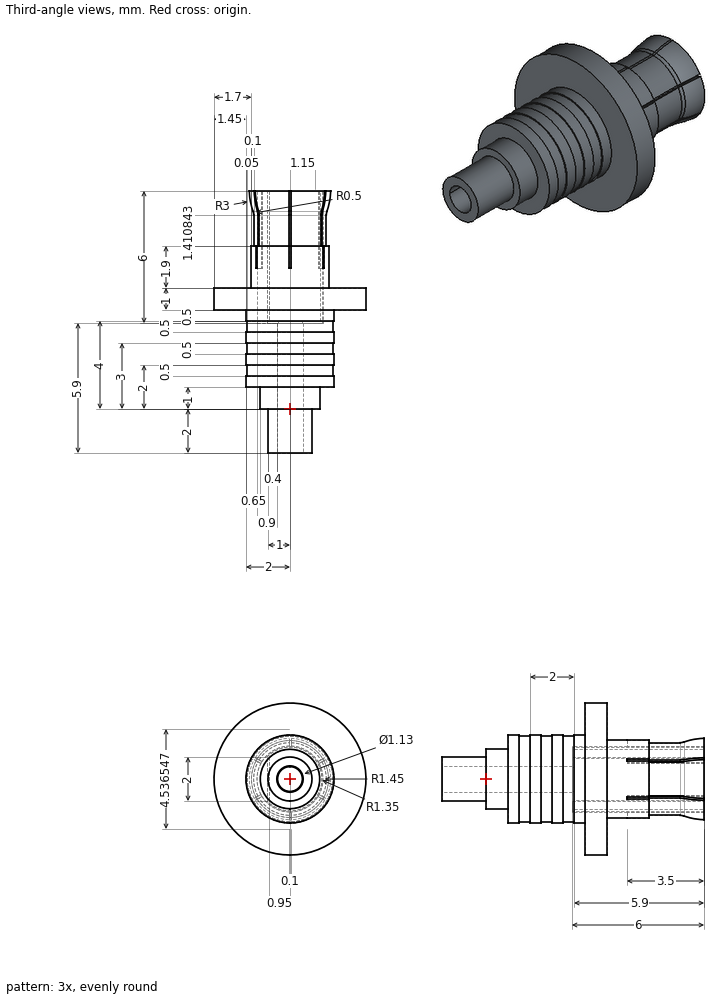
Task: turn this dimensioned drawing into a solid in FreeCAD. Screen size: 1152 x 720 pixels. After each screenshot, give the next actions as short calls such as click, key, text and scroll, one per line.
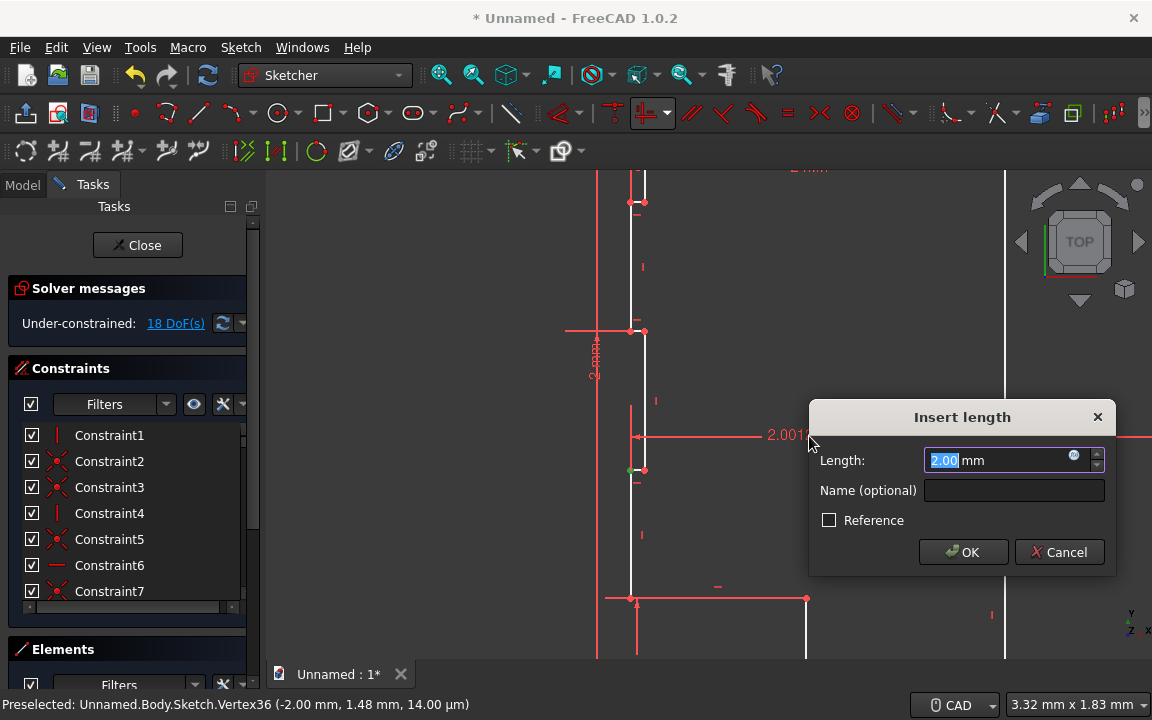
text(2)
key(Return)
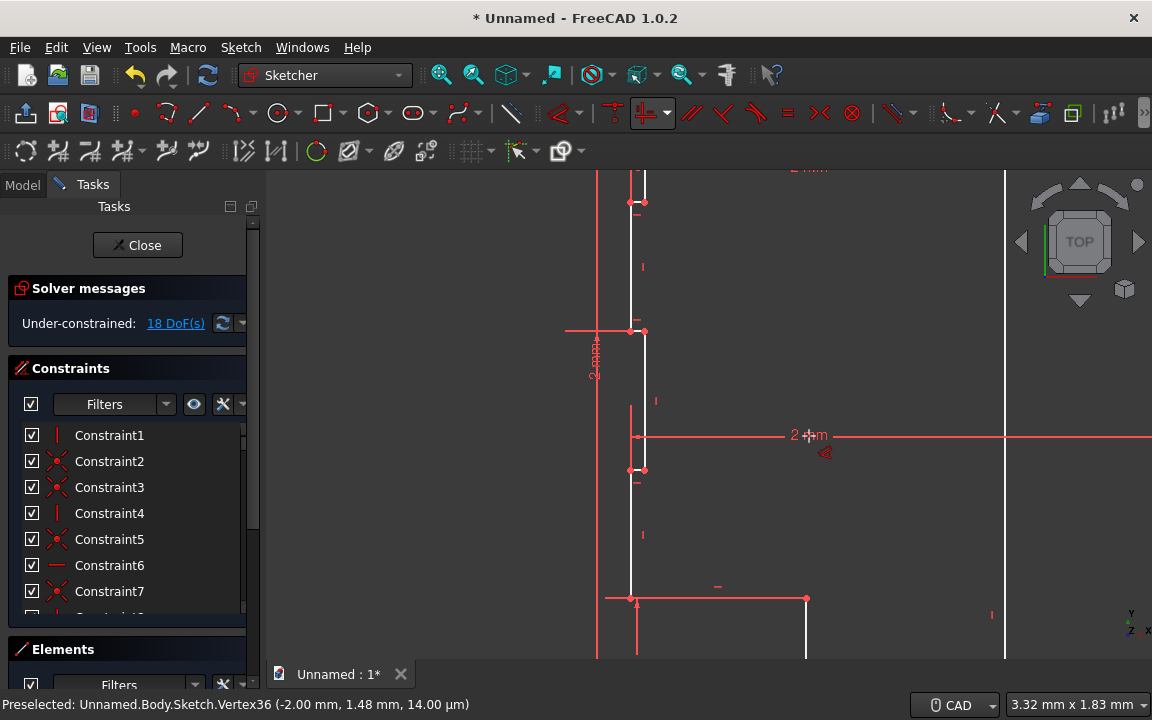
scroll(634, 475, down, 12)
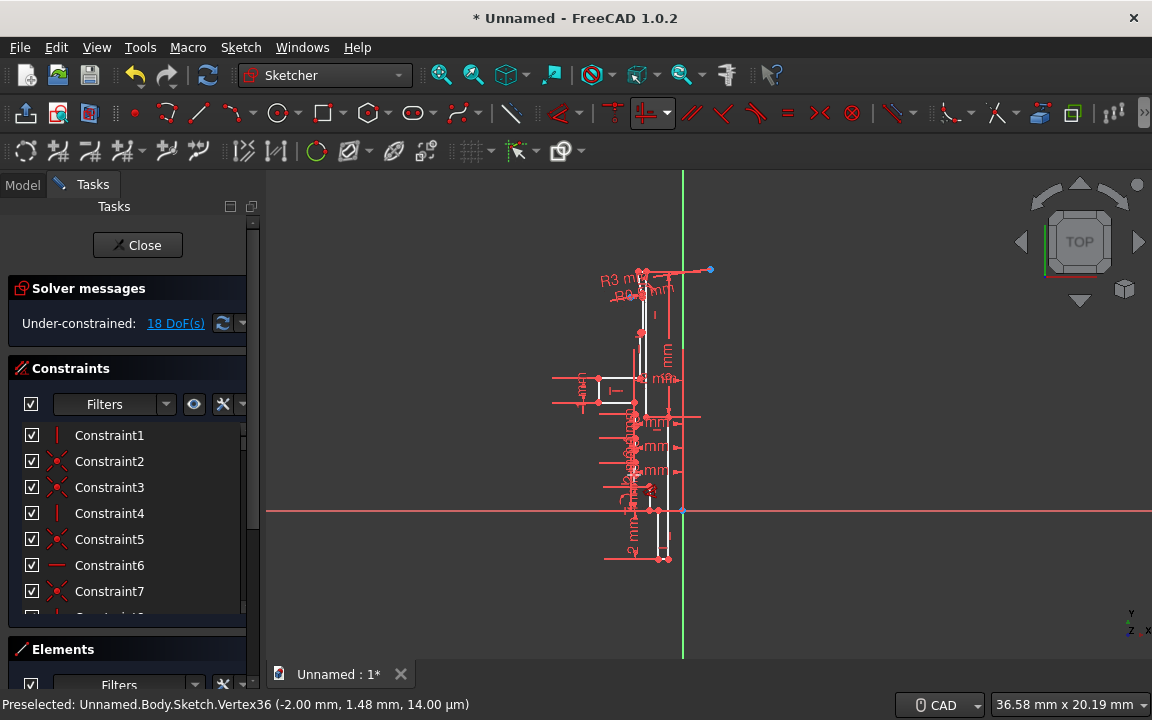
scroll(658, 511, up, 3)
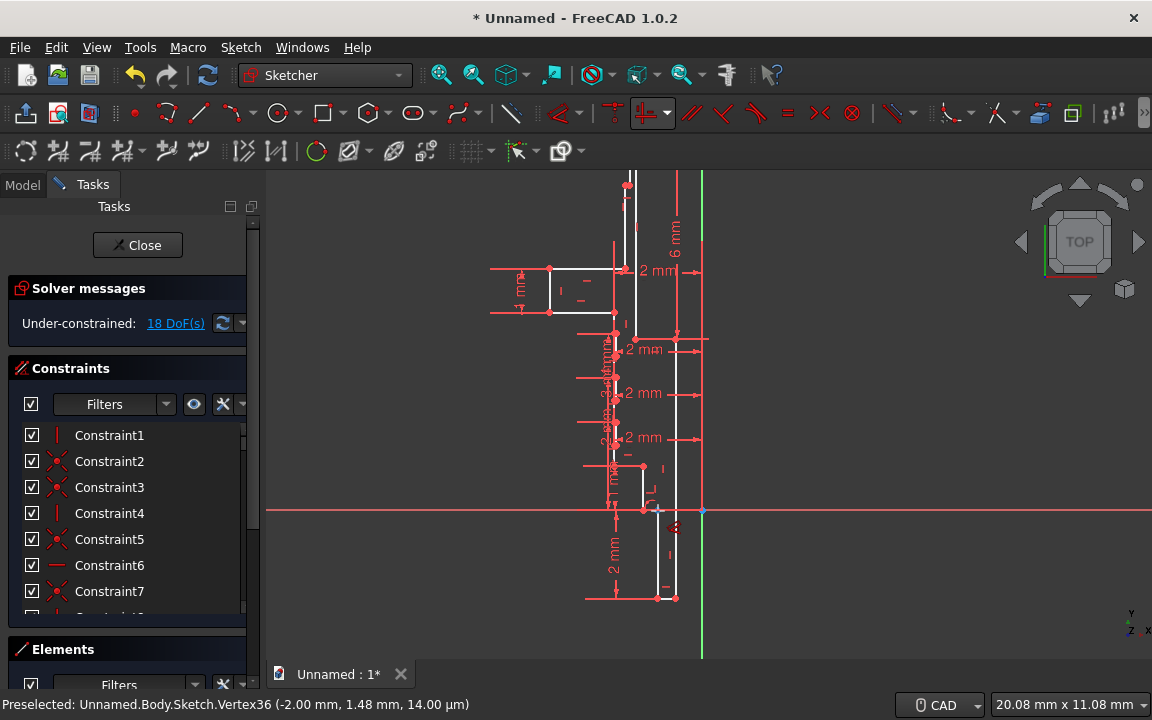
click(658, 510)
click(680, 616)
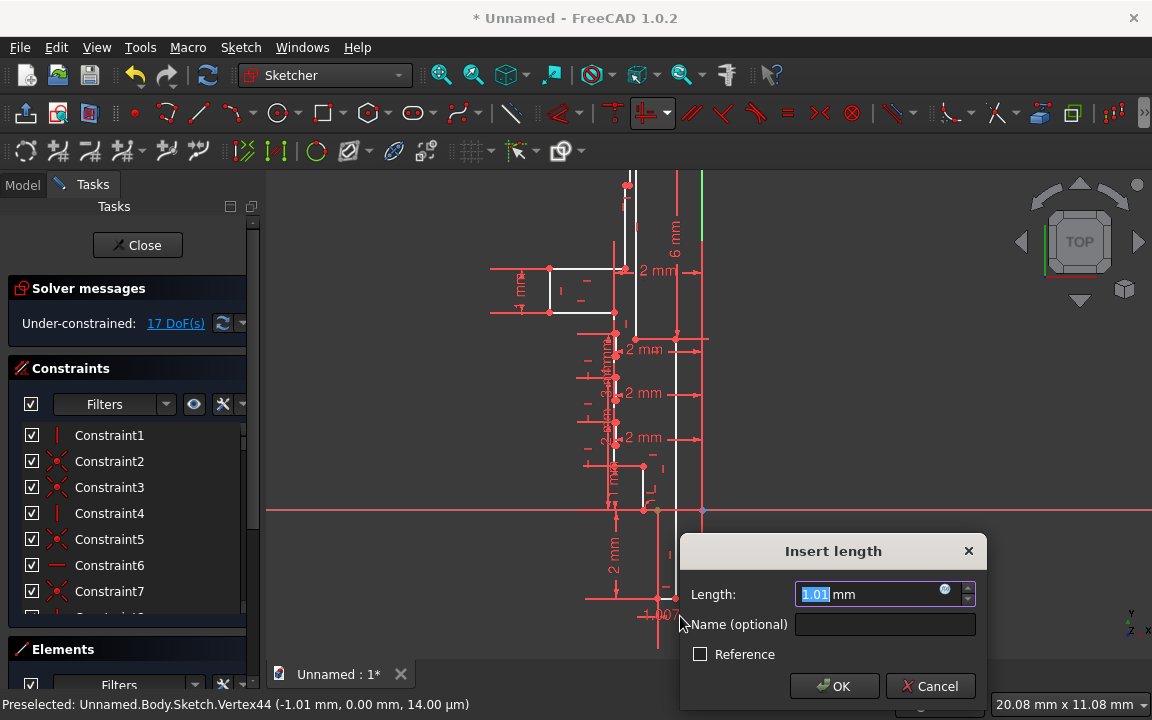
text(1)
key(Return)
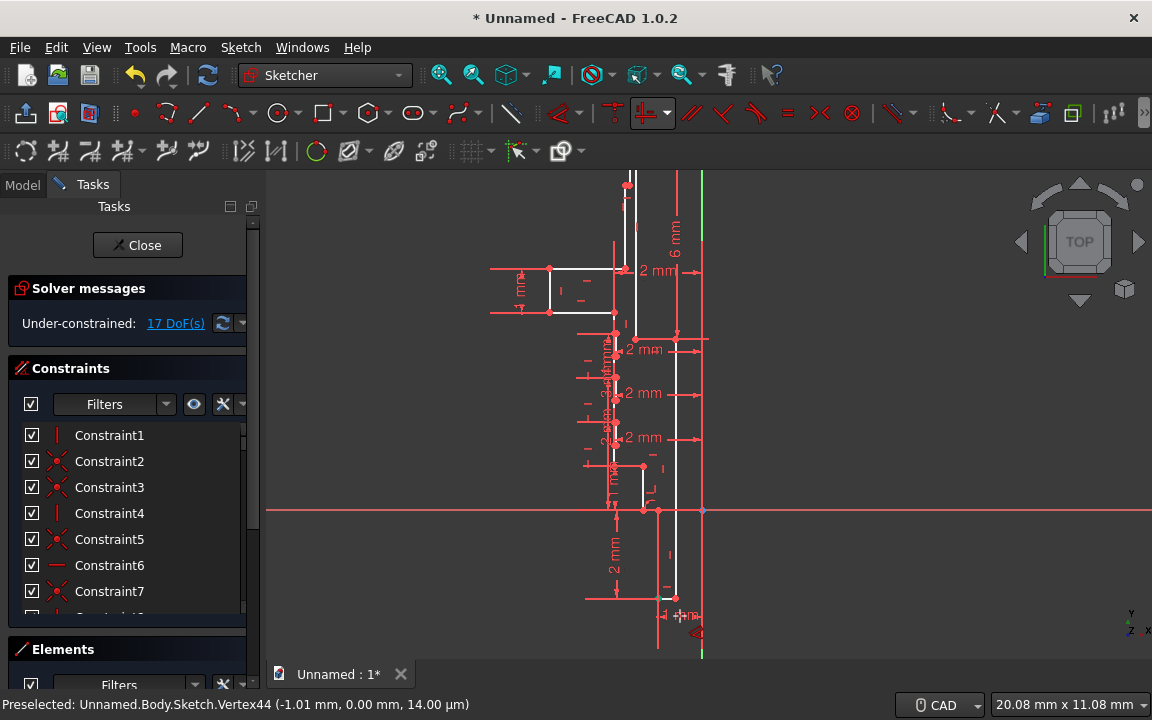
scroll(658, 510, down, 3)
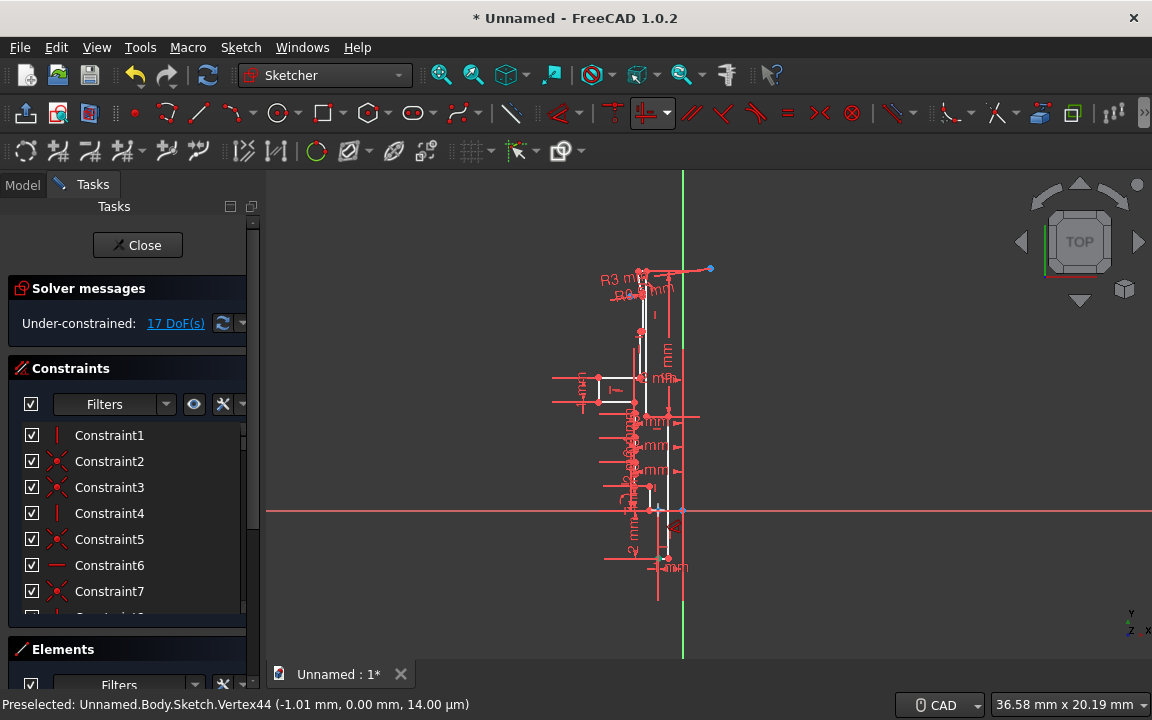
scroll(641, 332, up, 14)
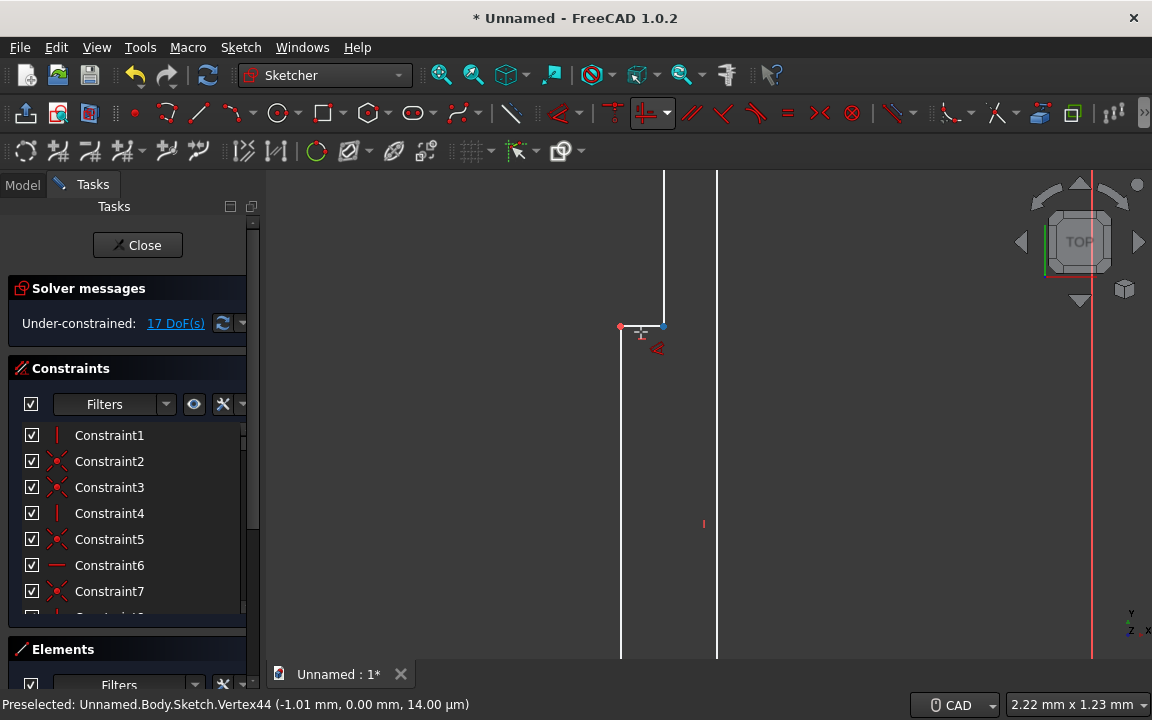
click(642, 326)
click(642, 292)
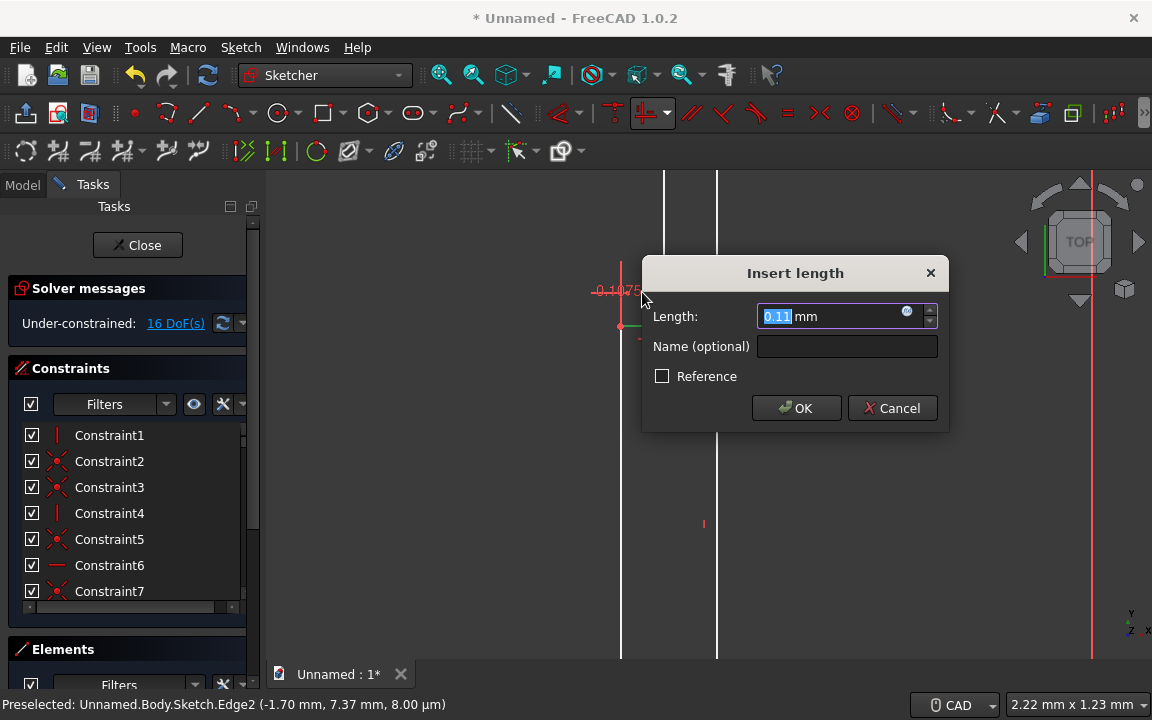
text(0.1)
key(Return)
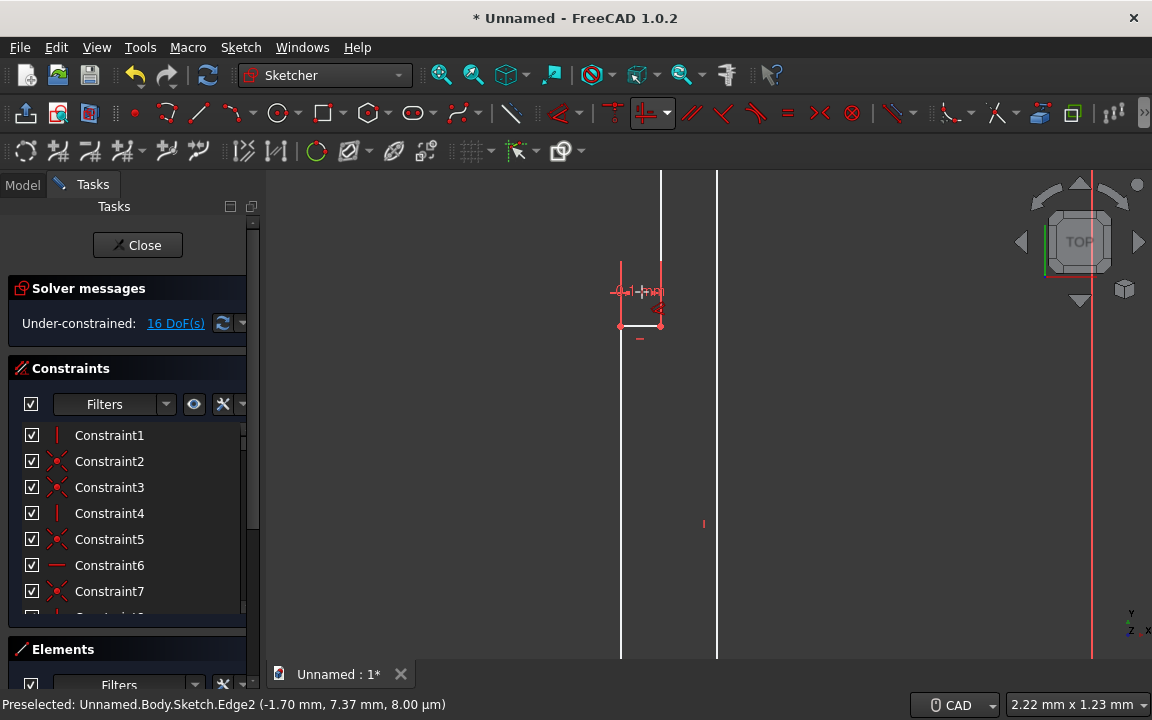
scroll(641, 332, down, 14)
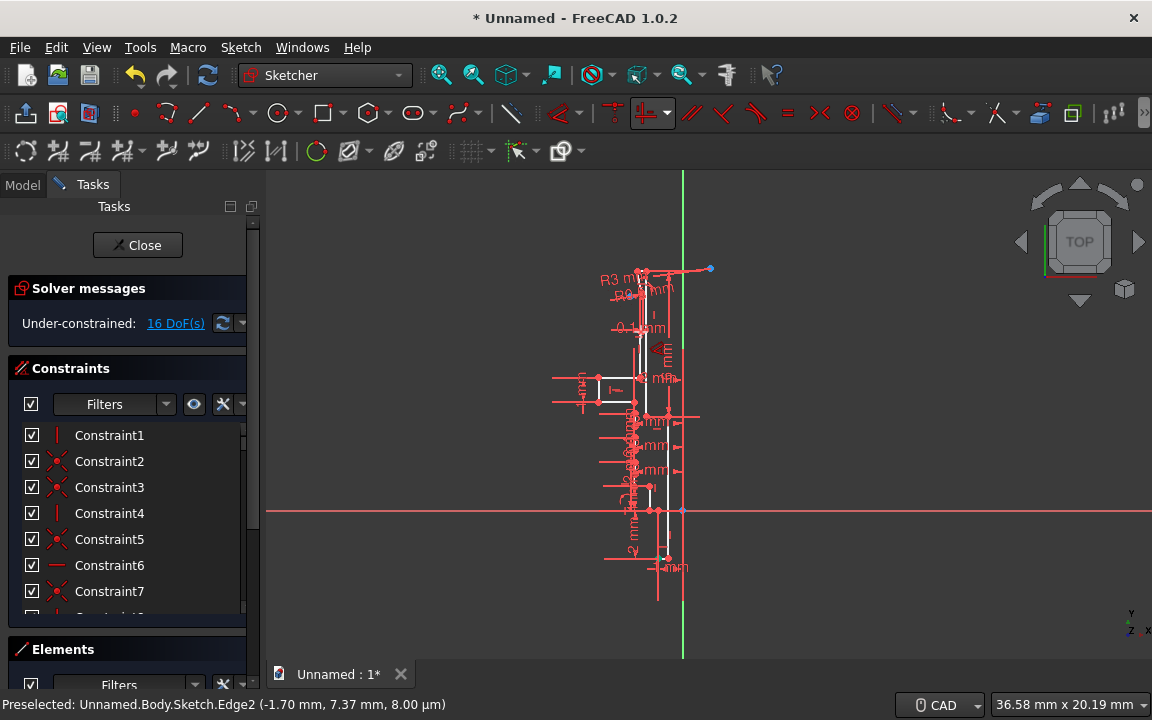
scroll(640, 346, up, 5)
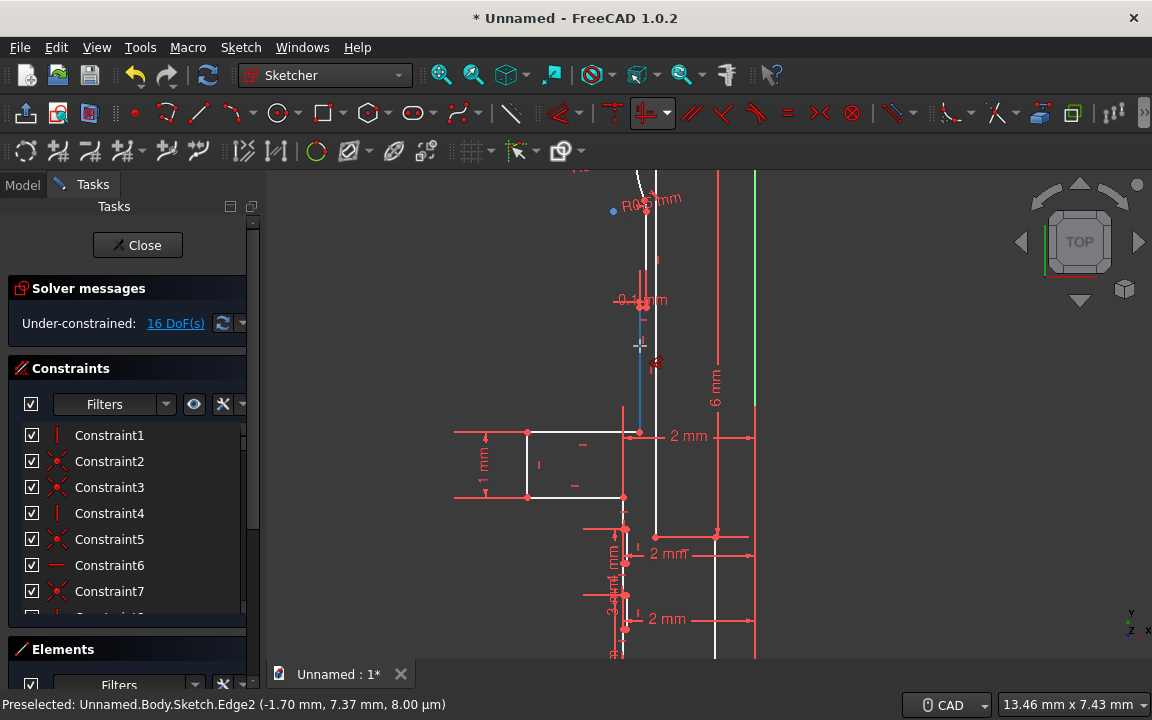
click(640, 345)
click(606, 370)